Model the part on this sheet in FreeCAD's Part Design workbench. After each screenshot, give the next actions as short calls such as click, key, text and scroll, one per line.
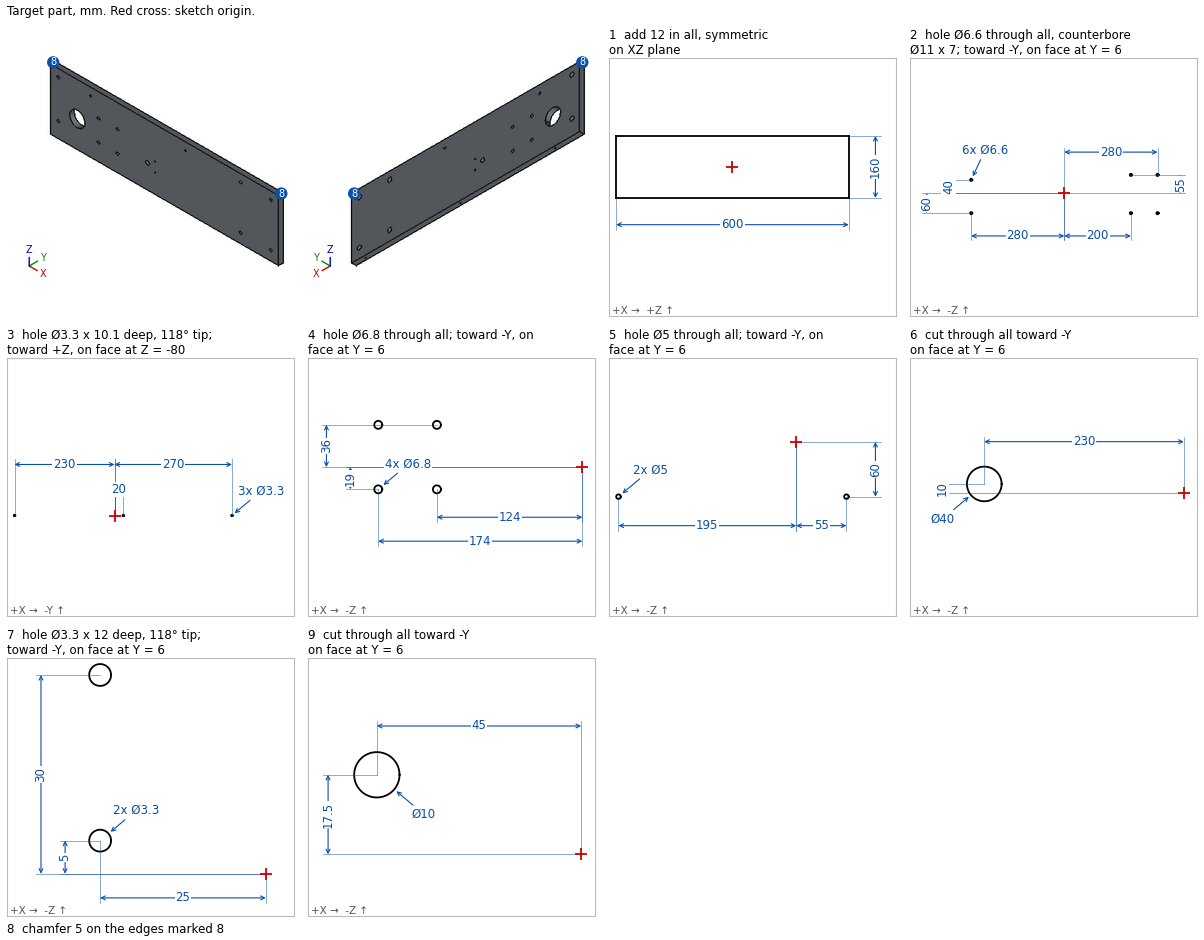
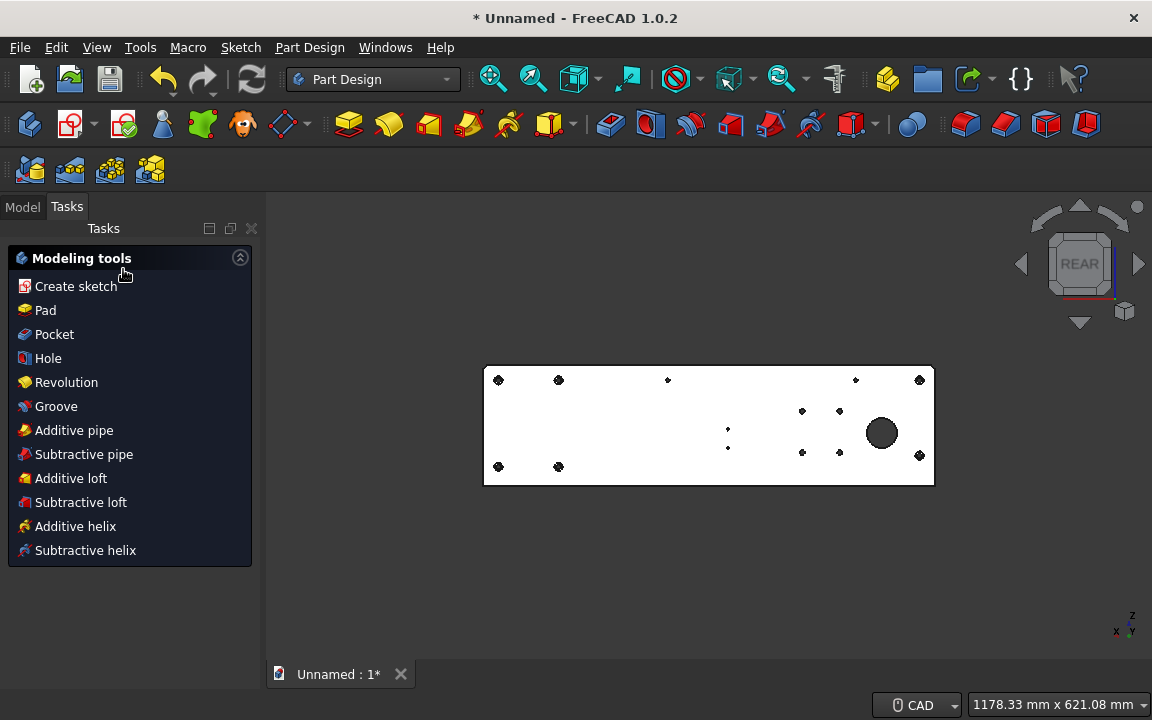
click(612, 124)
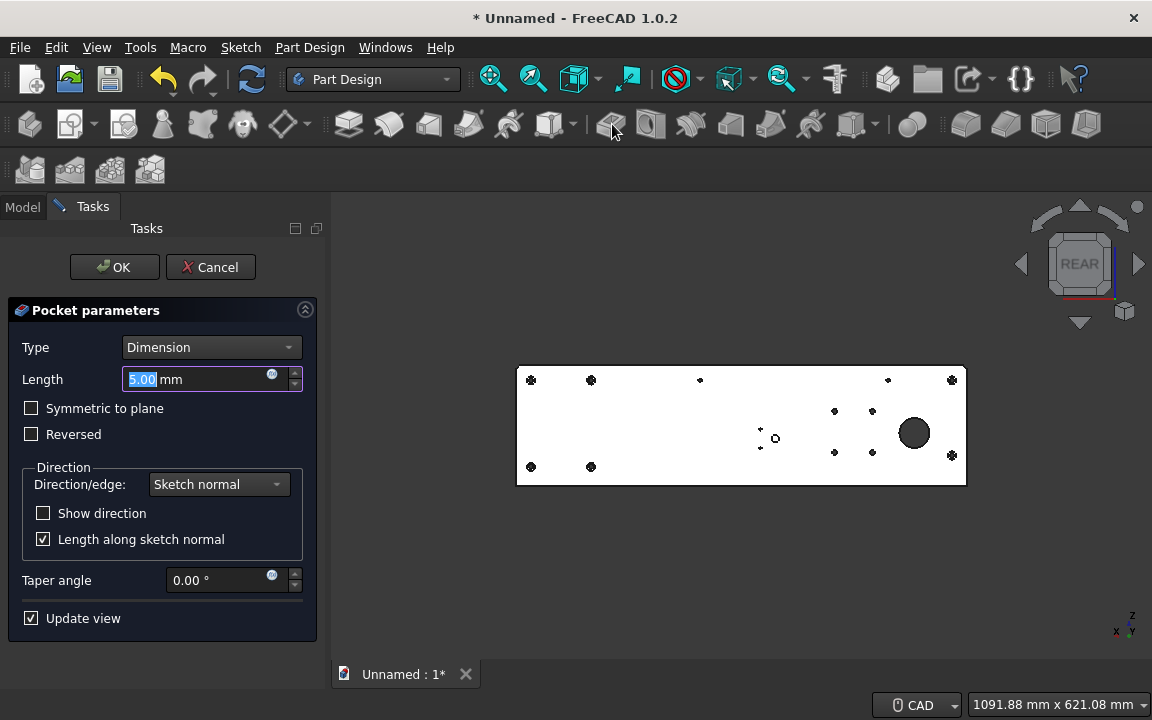
click(212, 348)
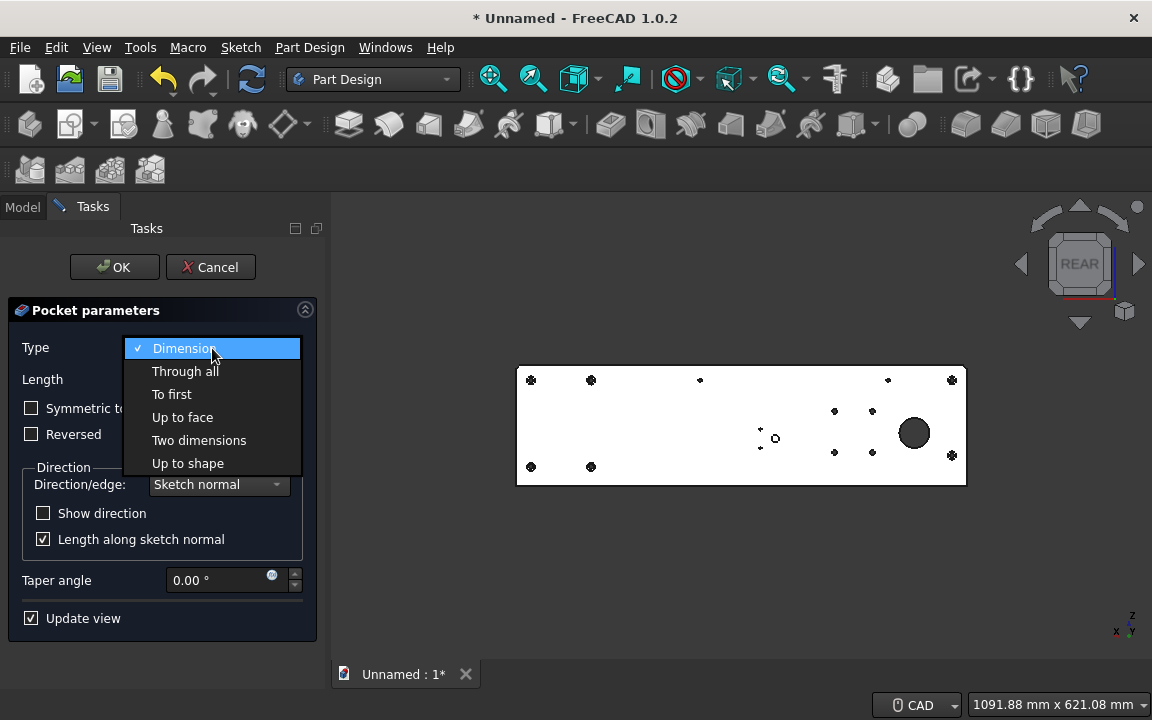
click(212, 372)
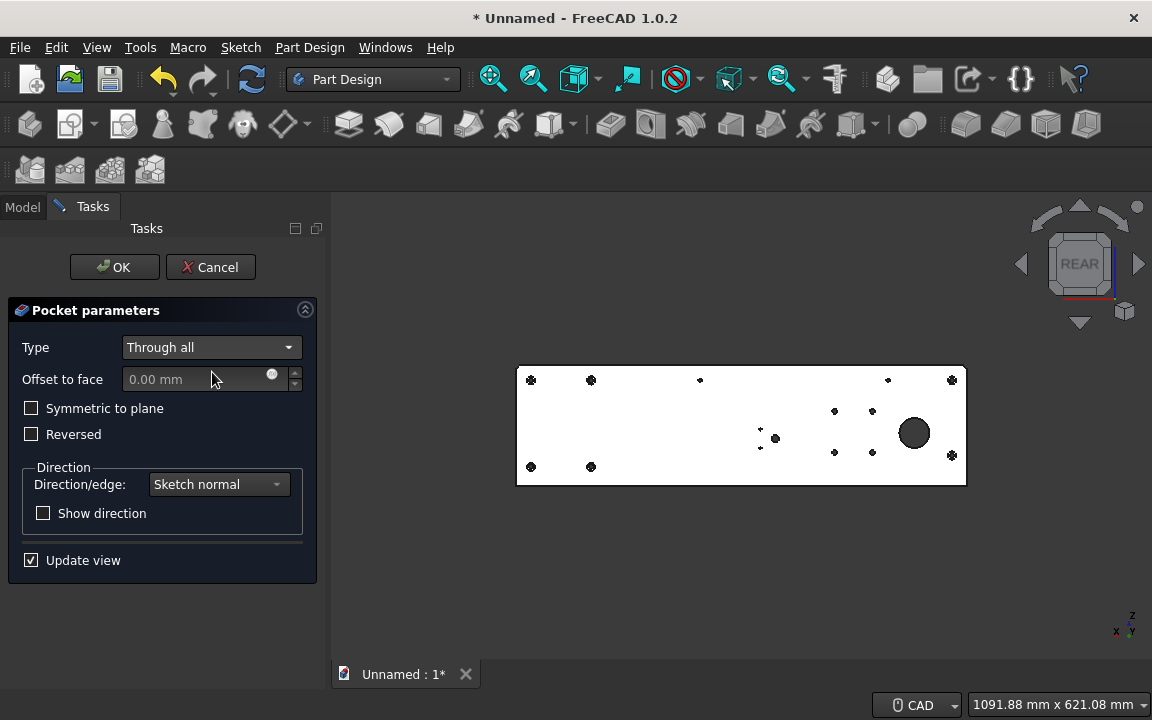
click(115, 267)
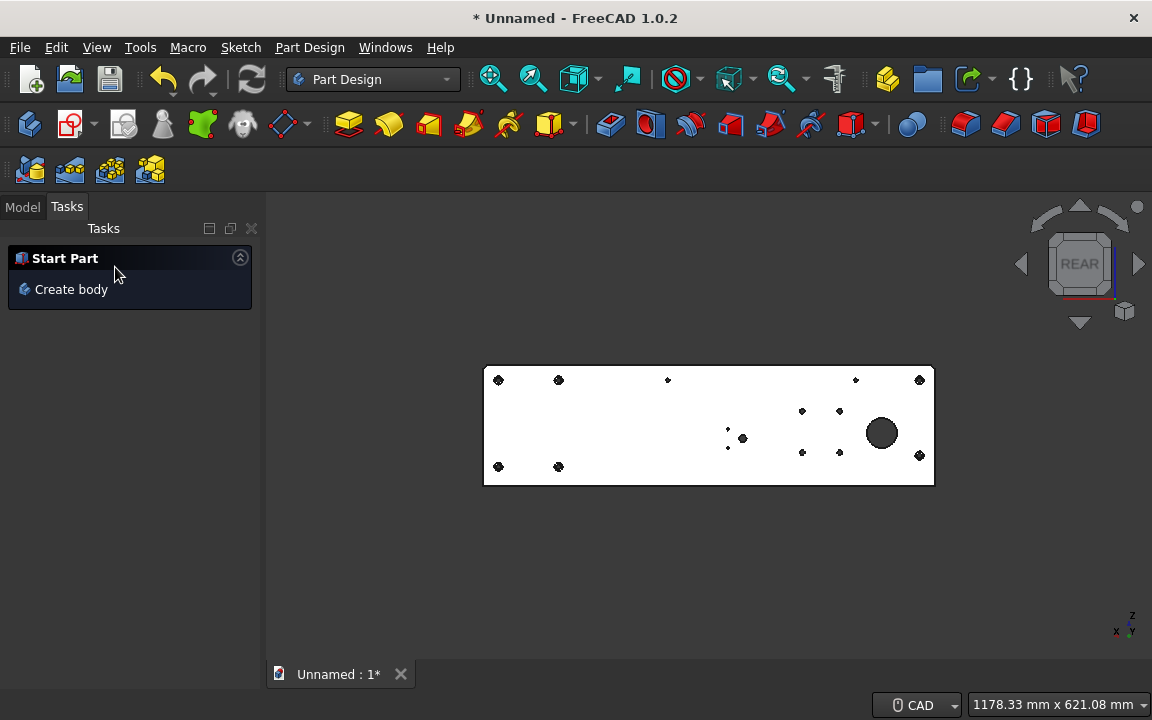
key(0)